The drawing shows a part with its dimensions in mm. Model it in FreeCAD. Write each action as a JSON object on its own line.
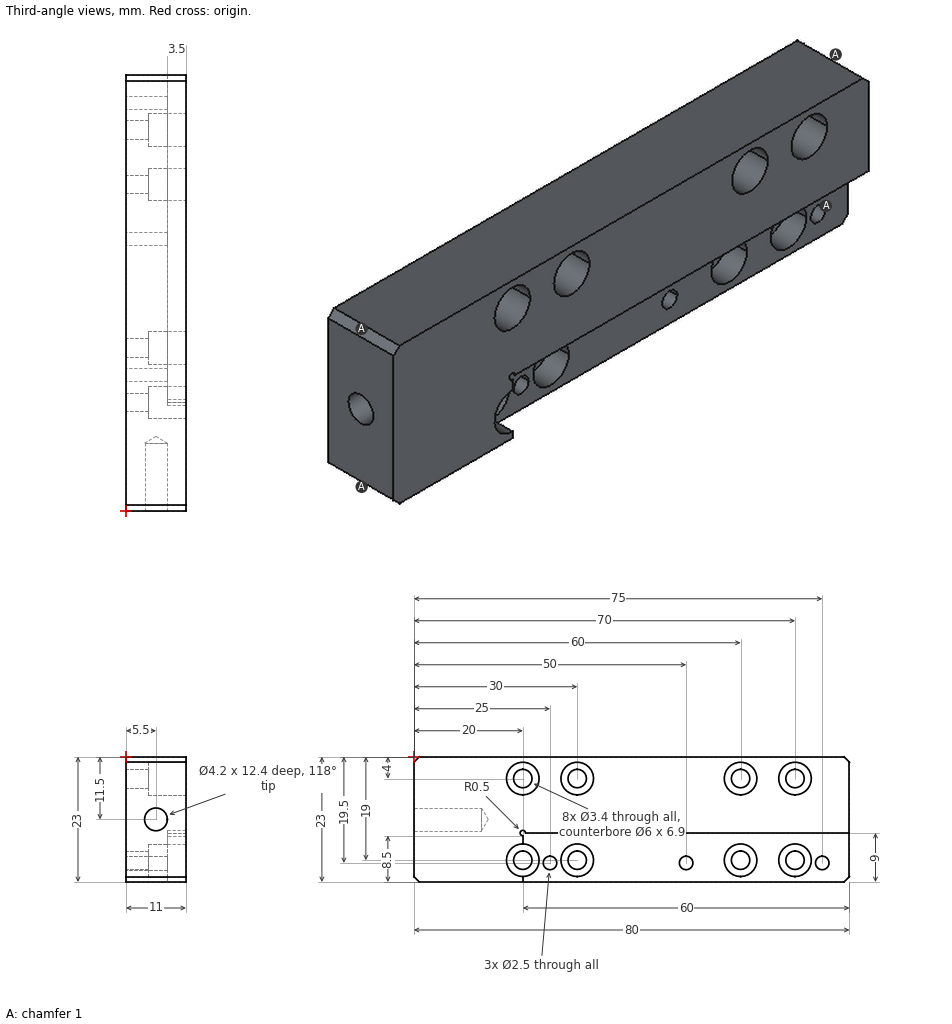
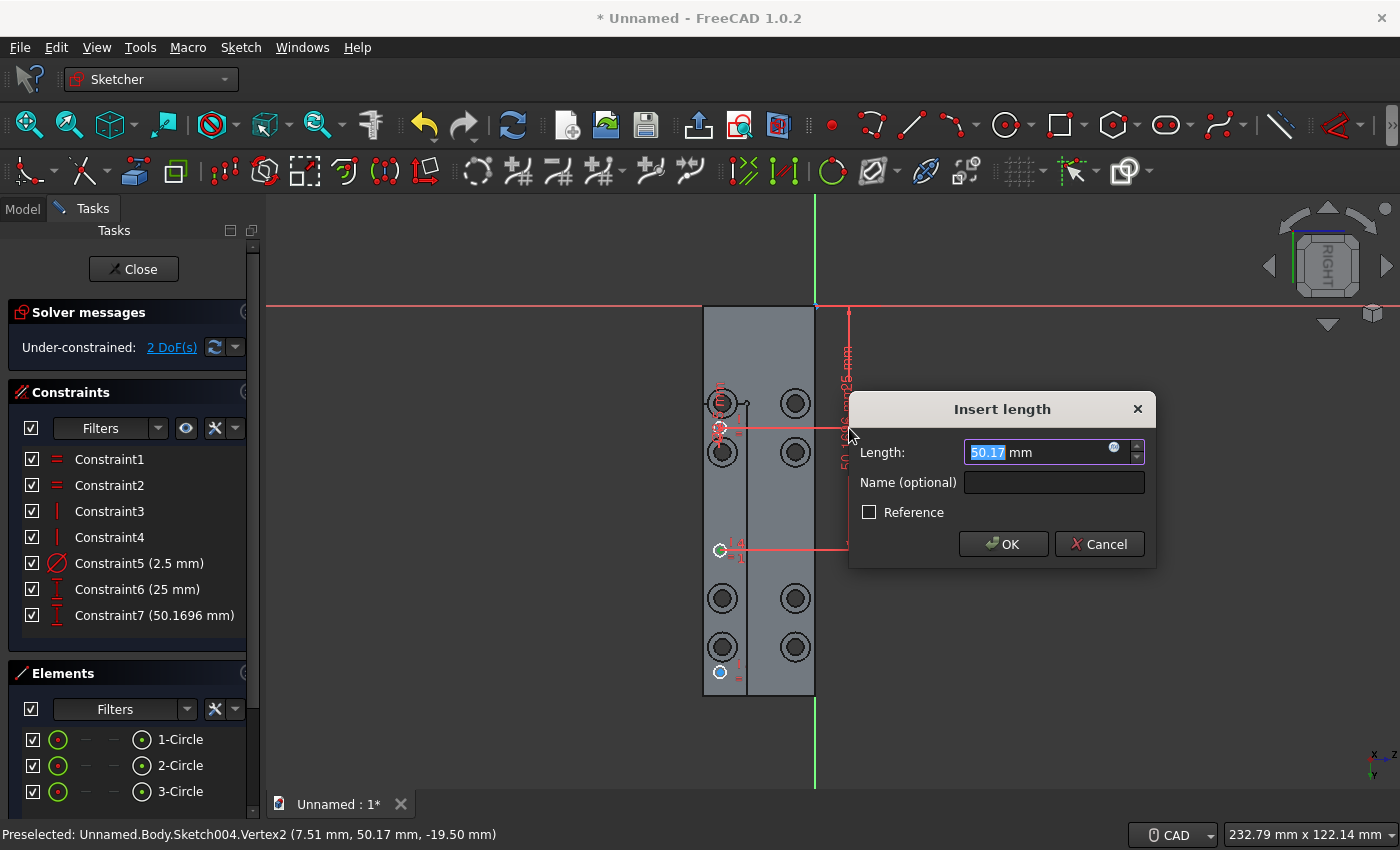
{"action": "type", "text": "50"}
{"action": "key", "text": "Return"}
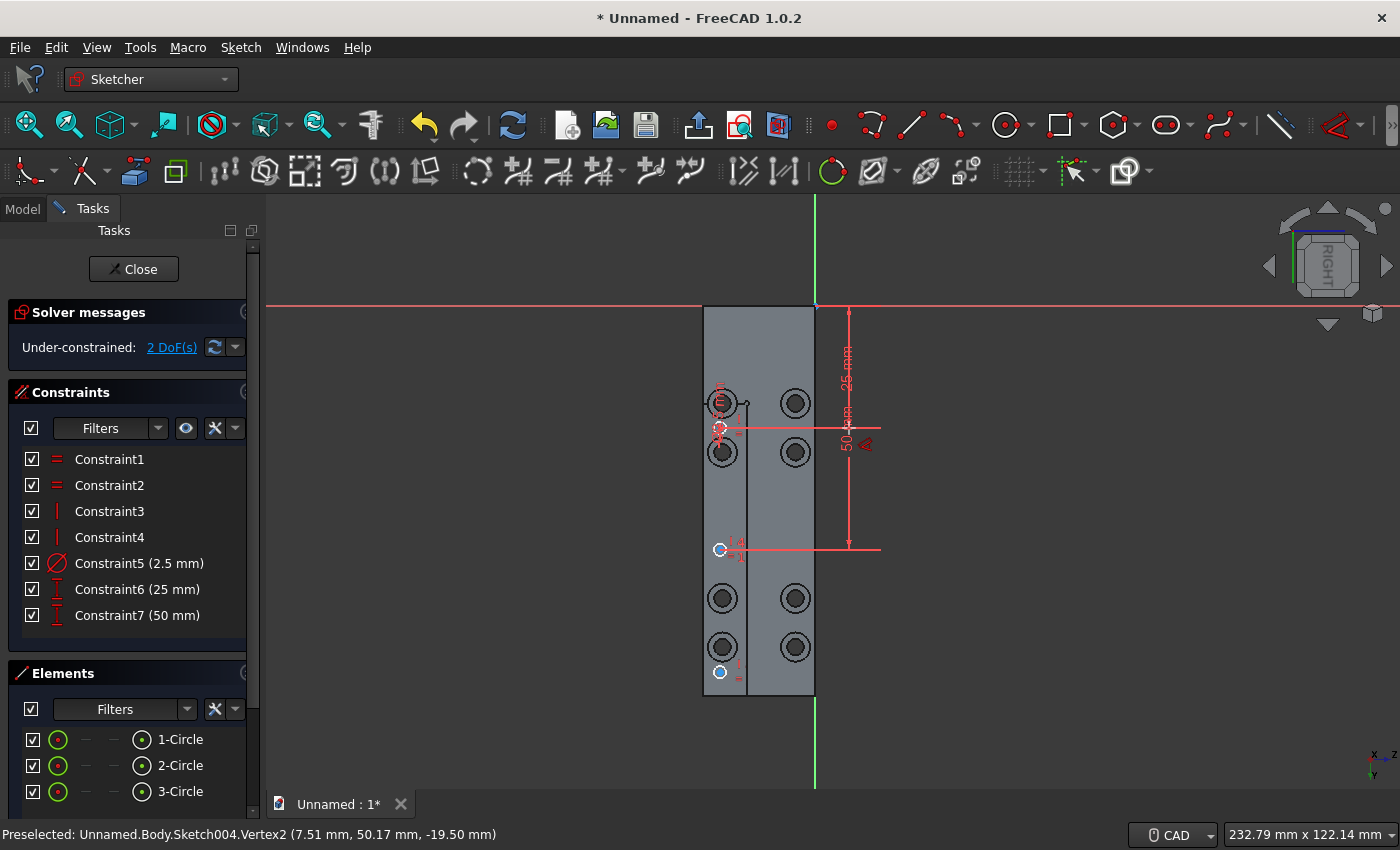
{"action": "left_click", "coordinate": [720, 672]}
{"action": "left_click", "coordinate": [849, 489]}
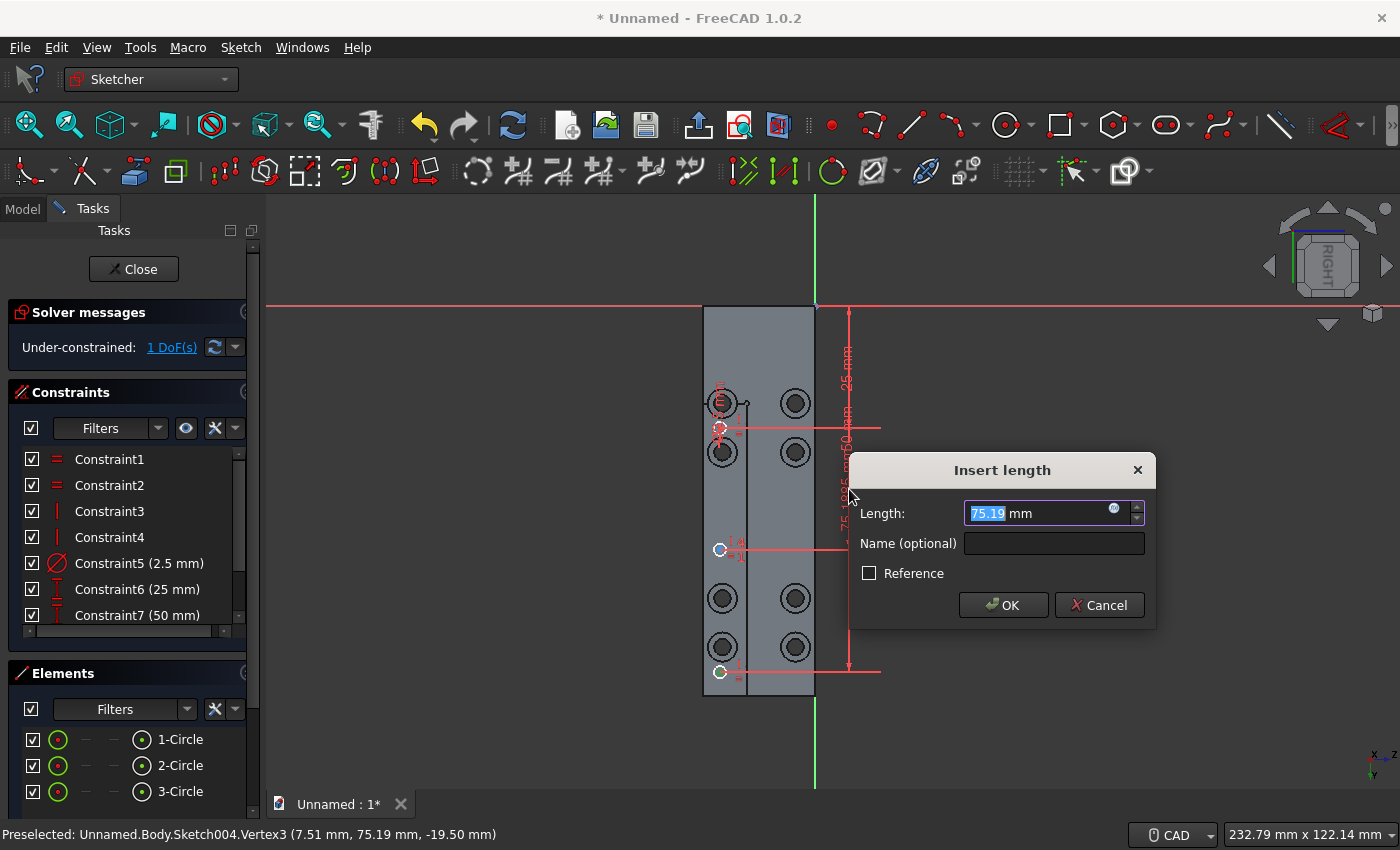
{"action": "type", "text": "75"}
{"action": "key", "text": "Return"}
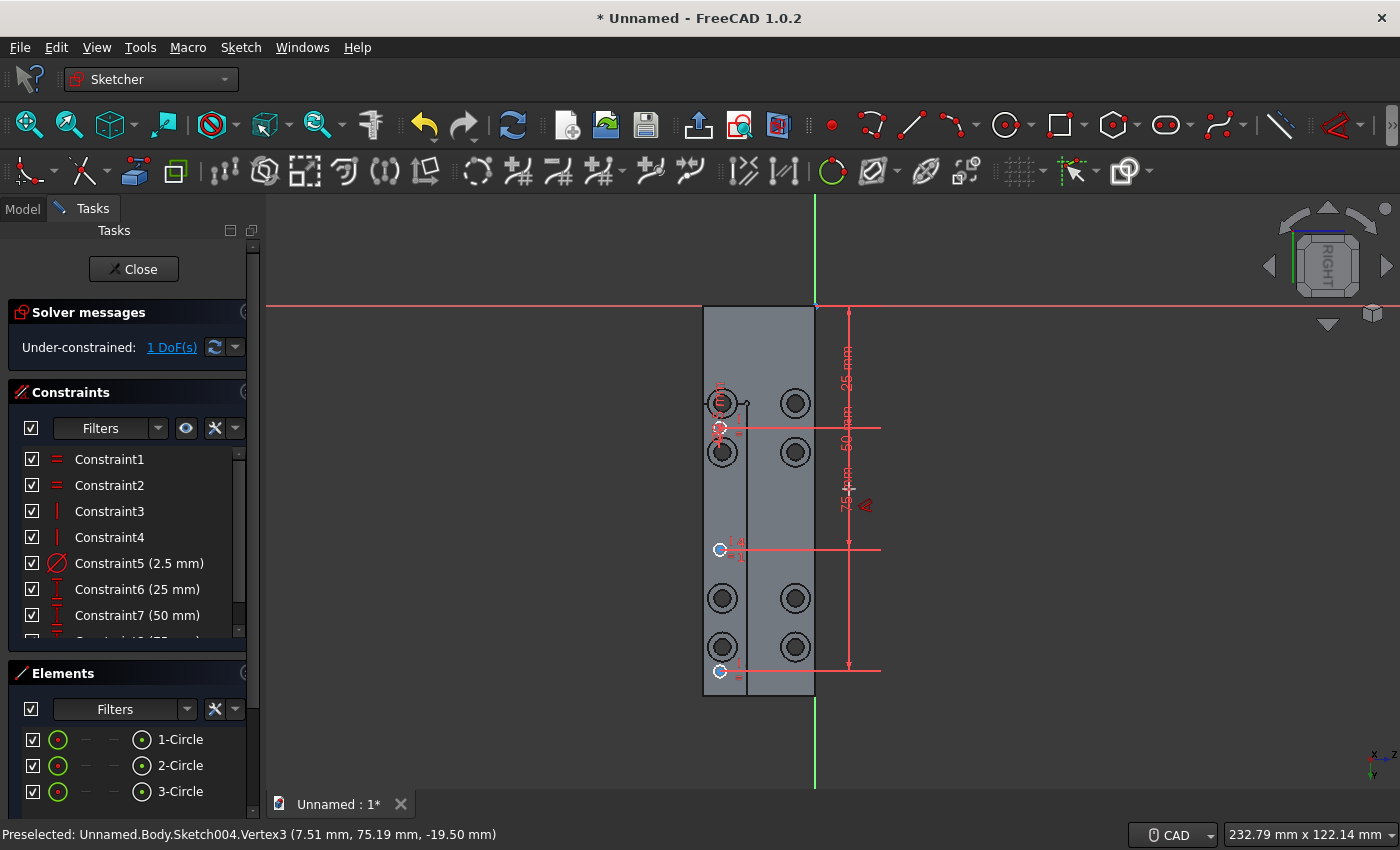
{"action": "left_click", "coordinate": [720, 428]}
{"action": "left_click", "coordinate": [768, 272]}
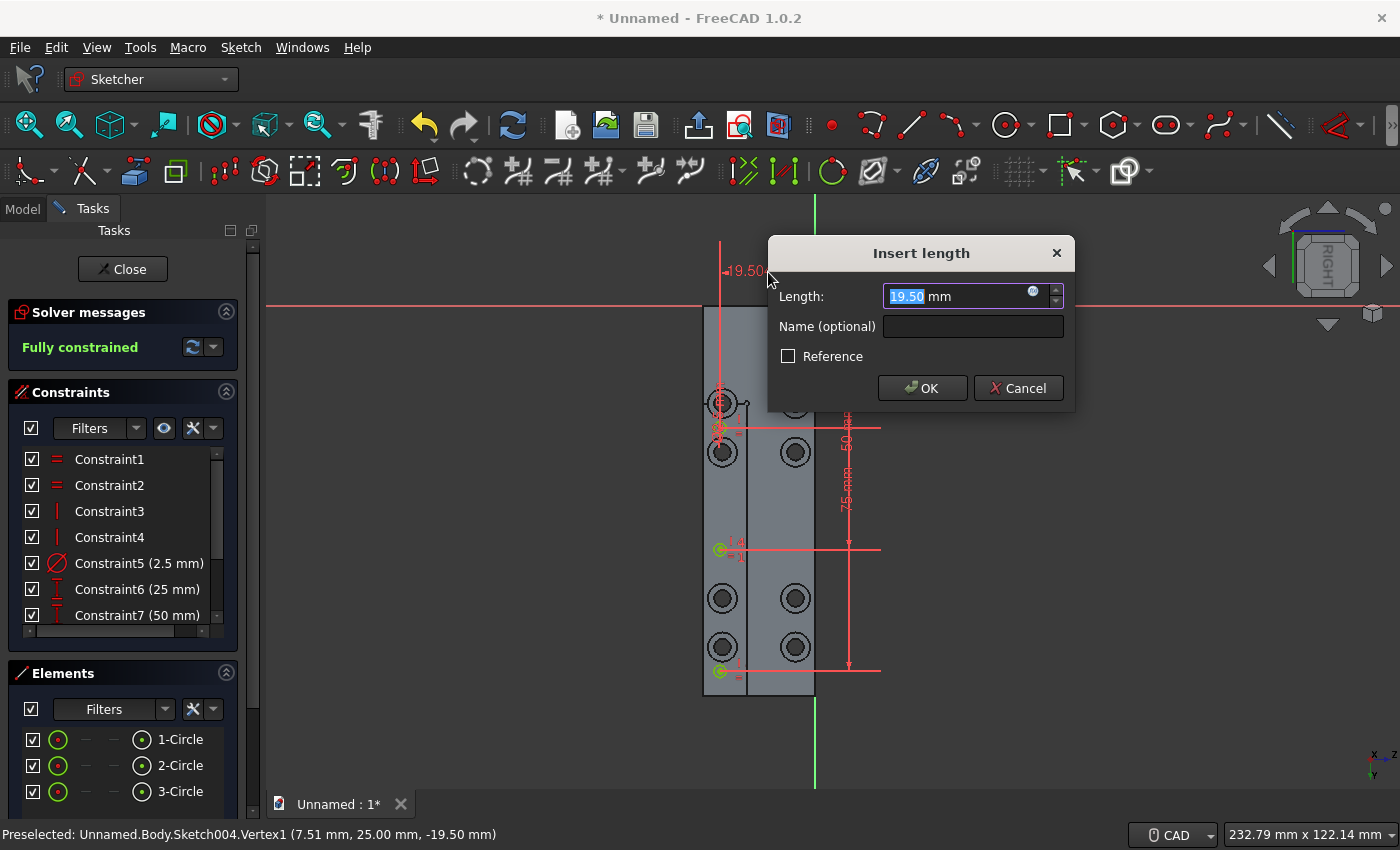
{"action": "type", "text": "19.5"}
{"action": "key", "text": "Return"}
{"action": "key", "text": "Escape"}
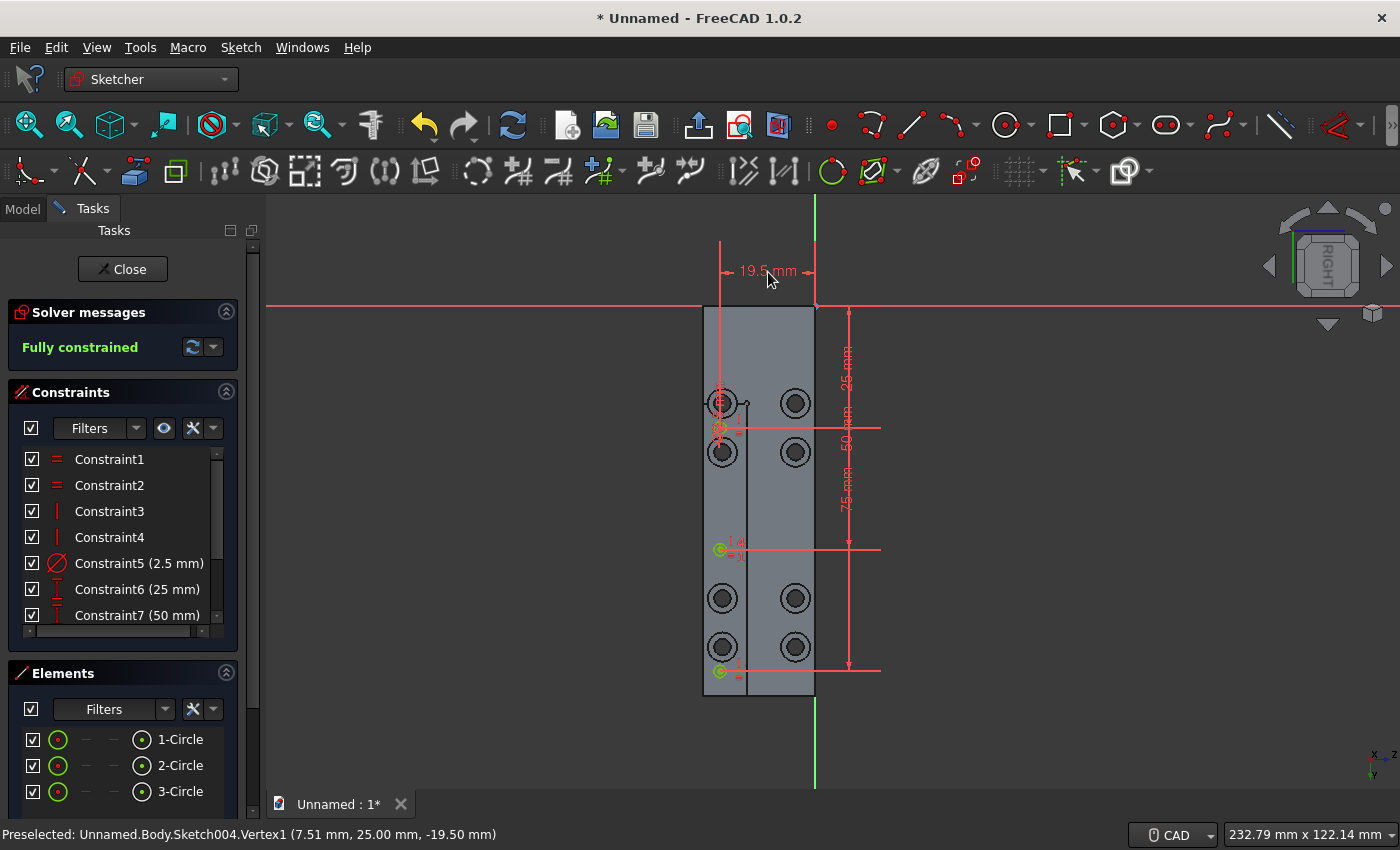
{"action": "left_click", "coordinate": [123, 269]}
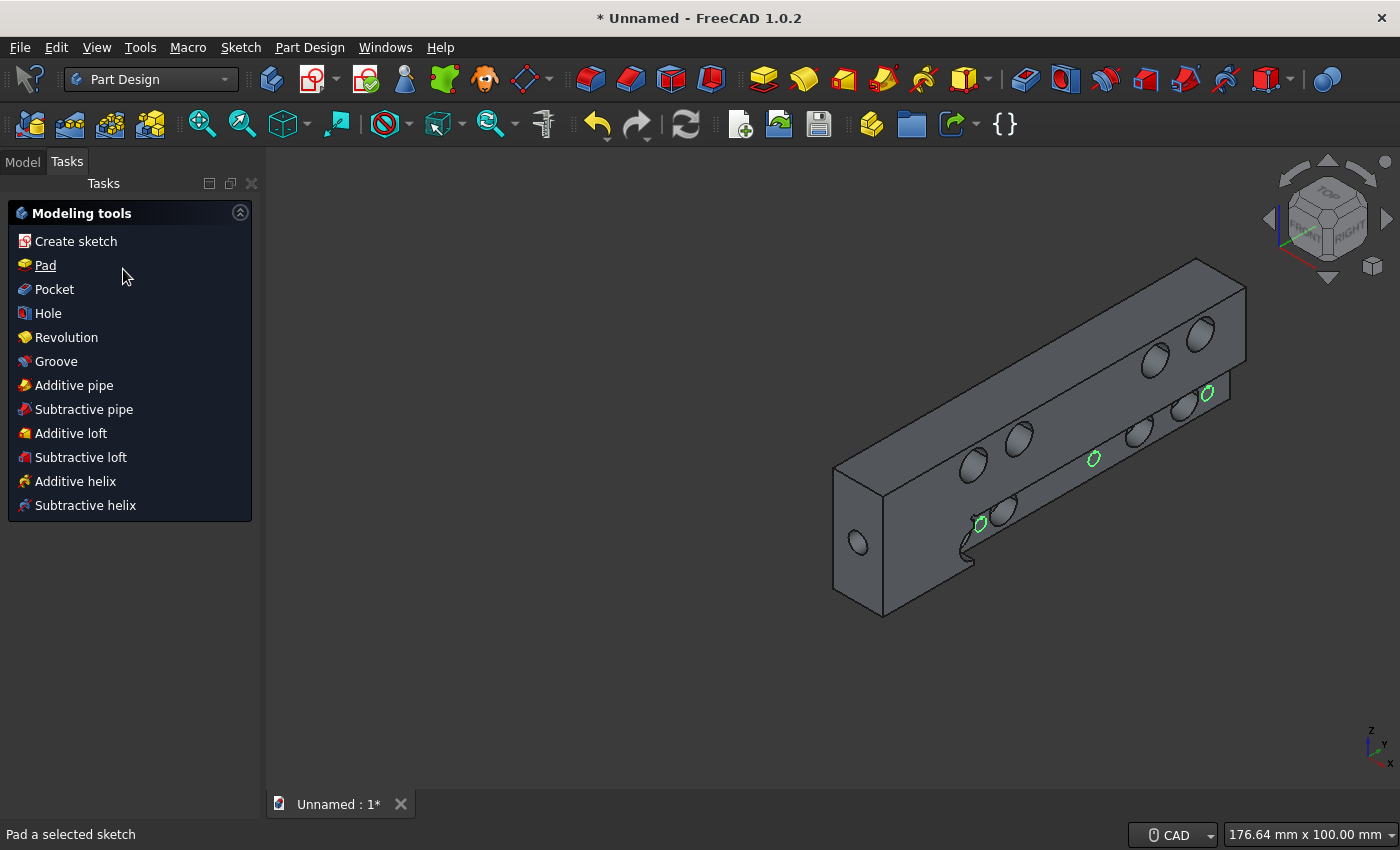
{"action": "left_click", "coordinate": [1066, 80]}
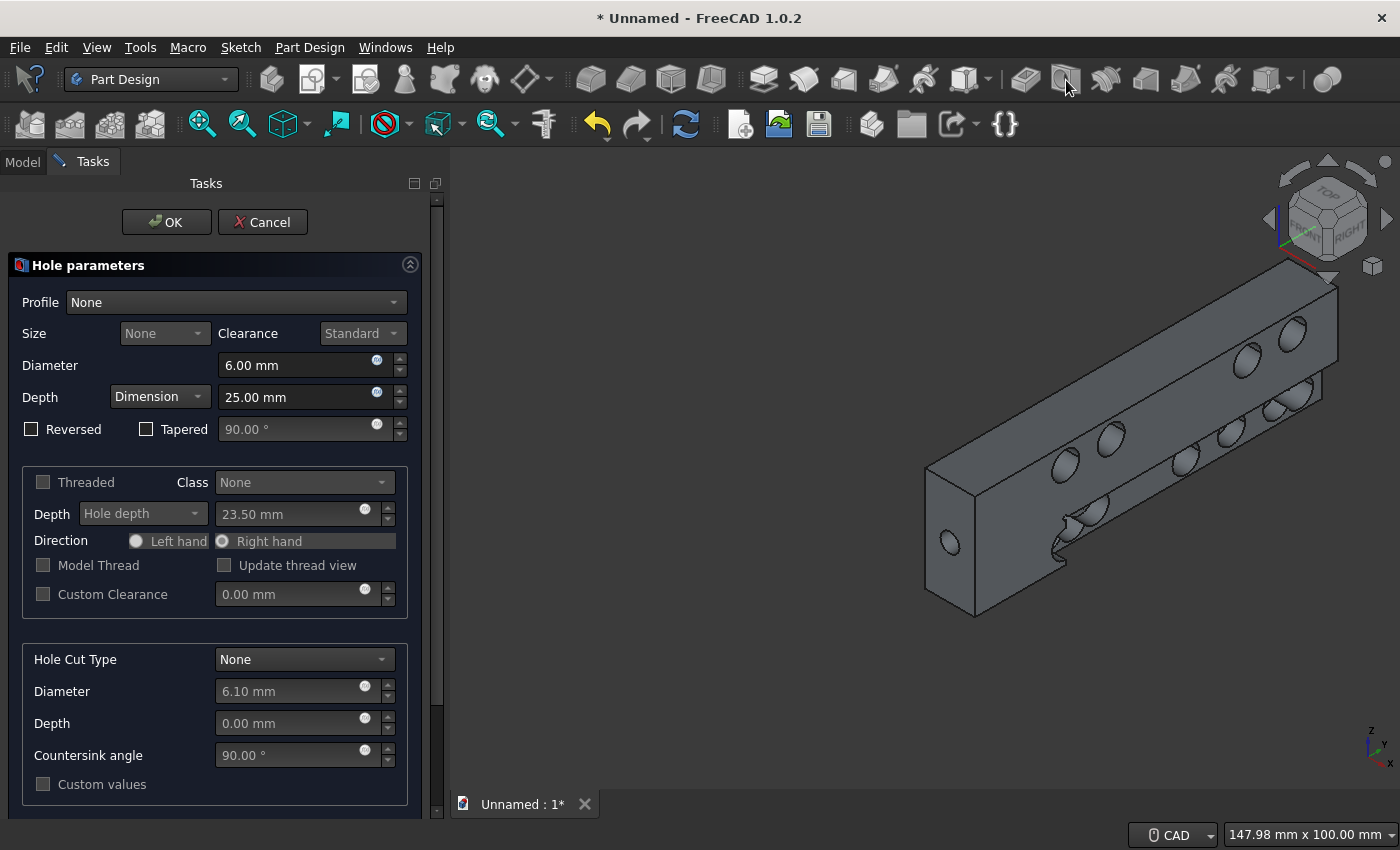
{"action": "triple_click", "coordinate": [305, 365]}